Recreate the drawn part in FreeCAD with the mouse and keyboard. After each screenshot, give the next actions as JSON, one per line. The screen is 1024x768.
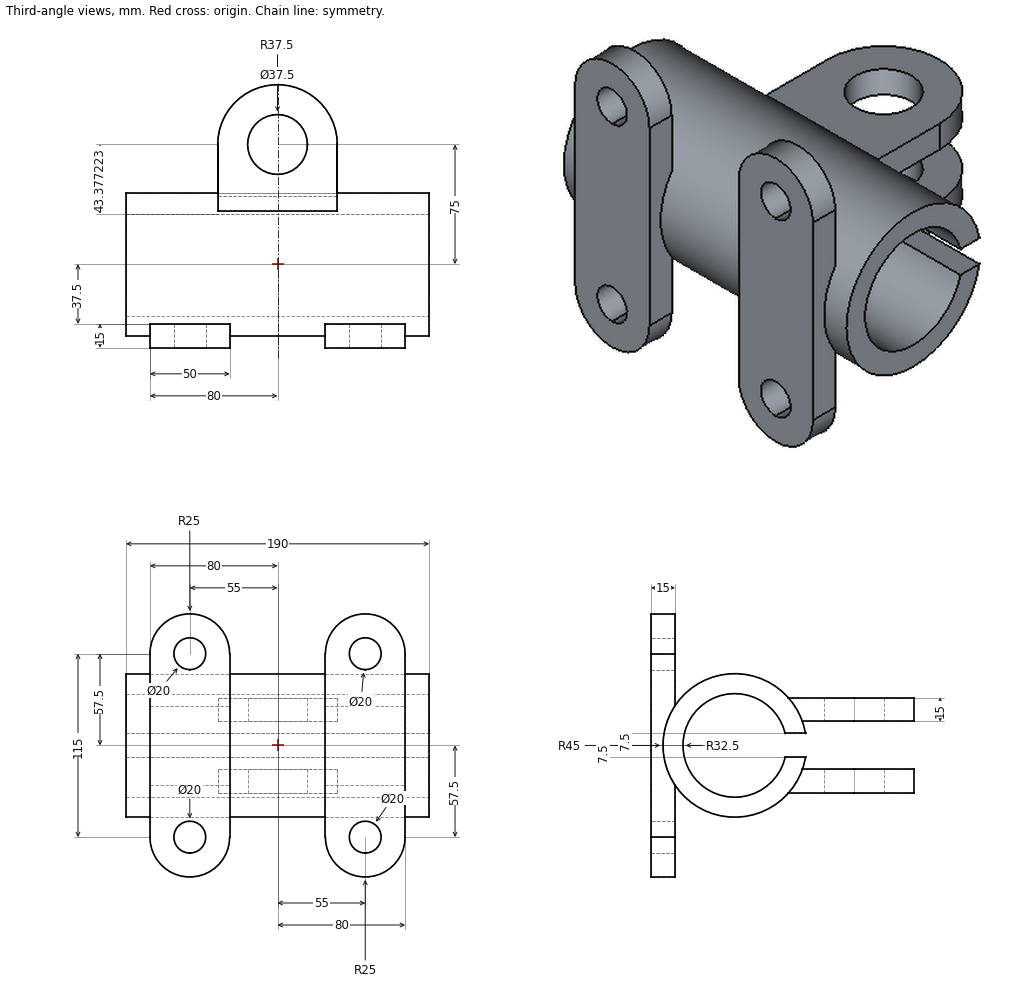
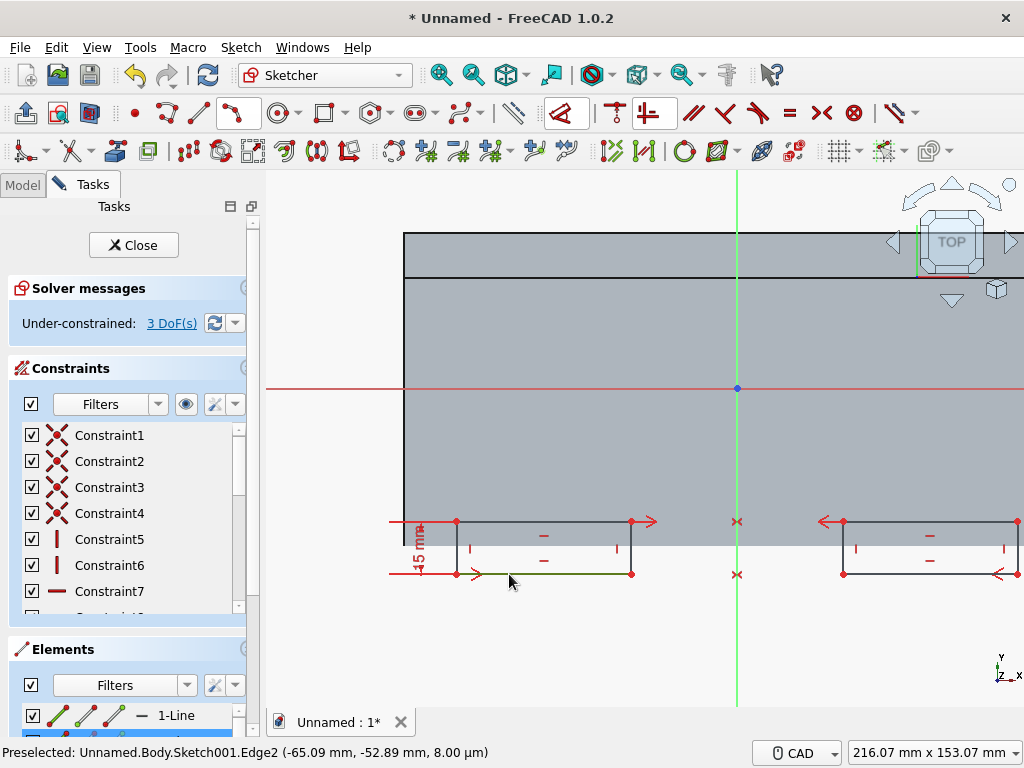
{"action": "left_click", "coordinate": [584, 114]}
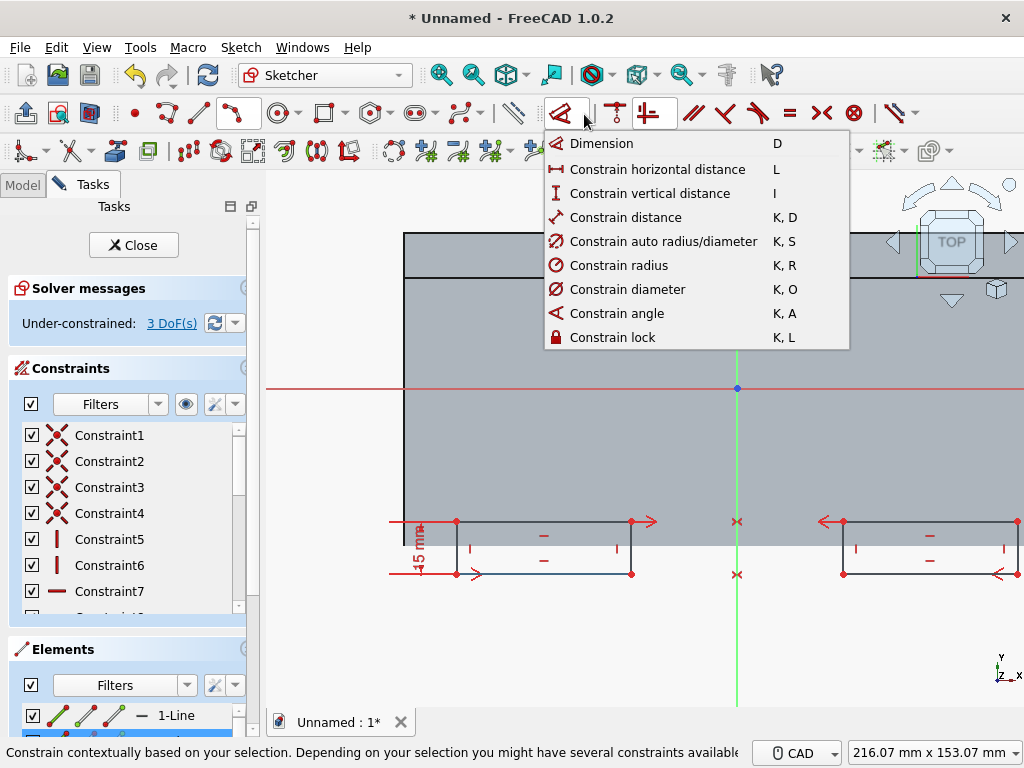
{"action": "left_click", "coordinate": [697, 169]}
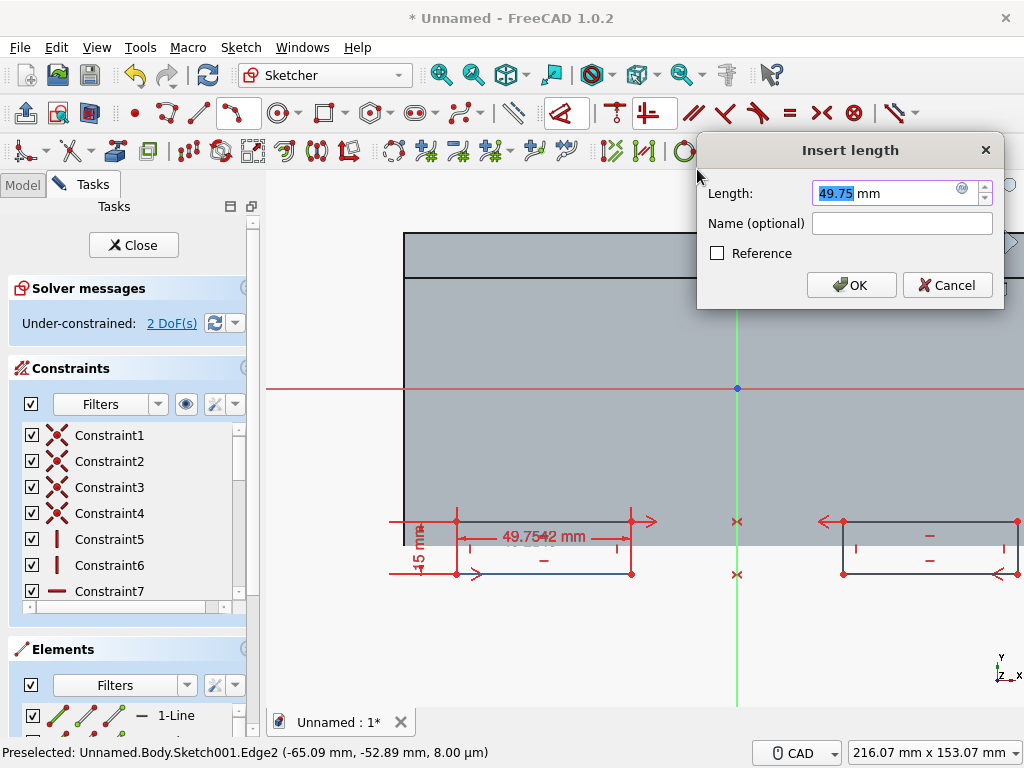
{"action": "type", "text": "50"}
{"action": "key", "text": "Return"}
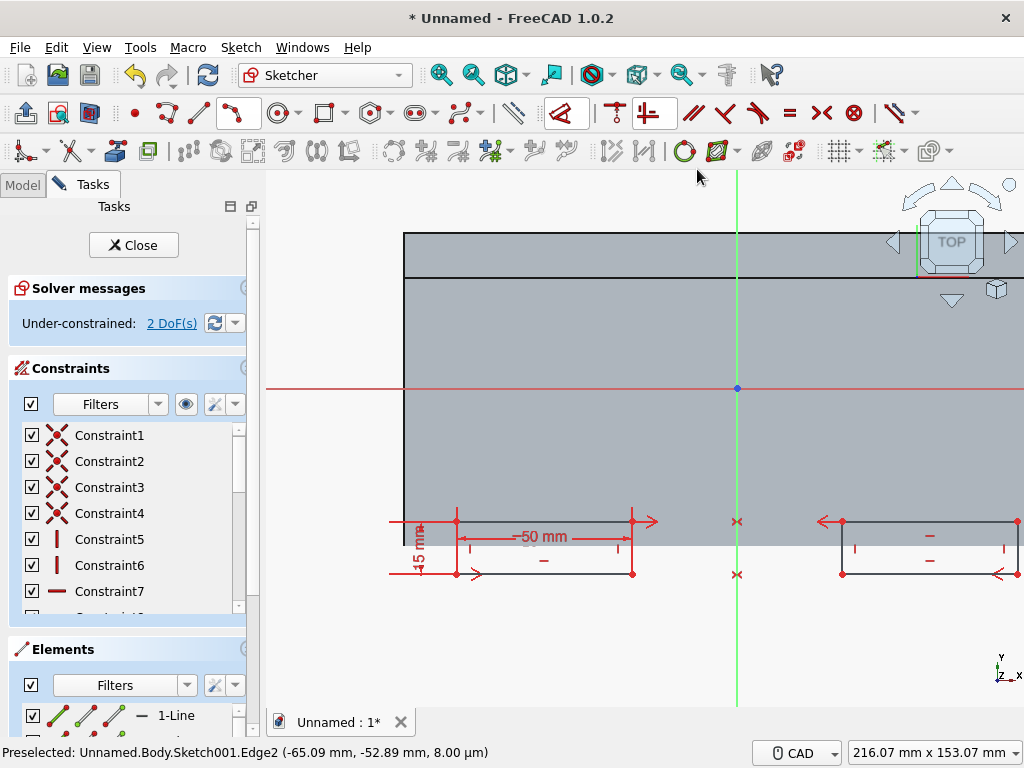
{"action": "left_click", "coordinate": [457, 522]}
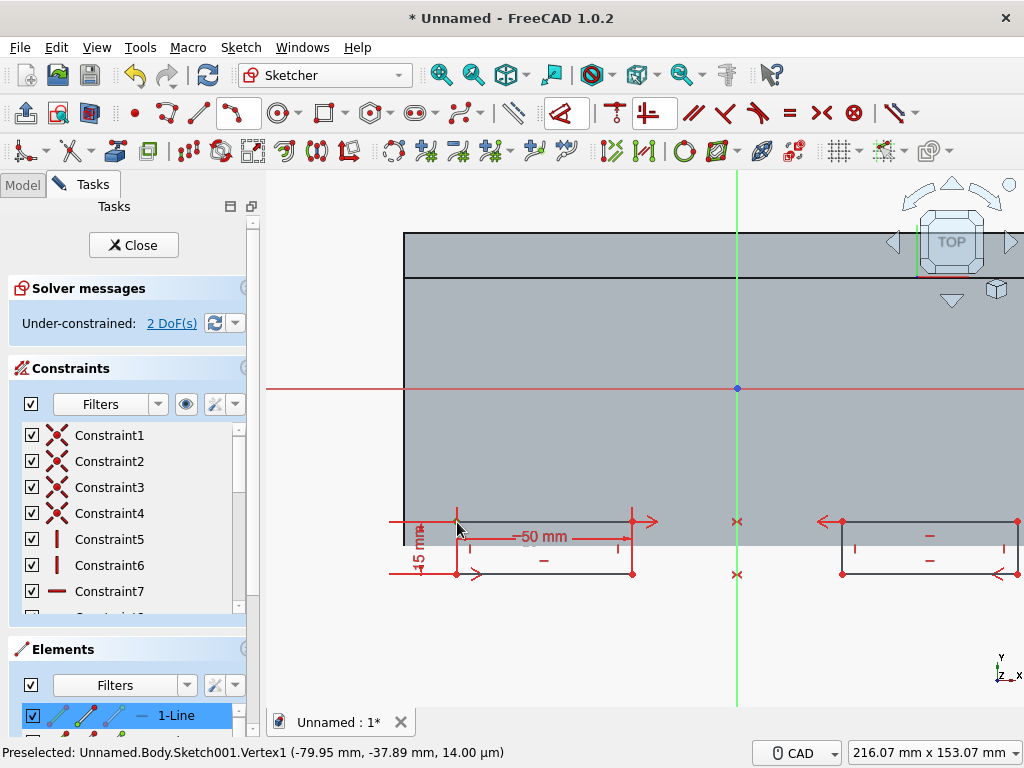
{"action": "left_click", "coordinate": [584, 114]}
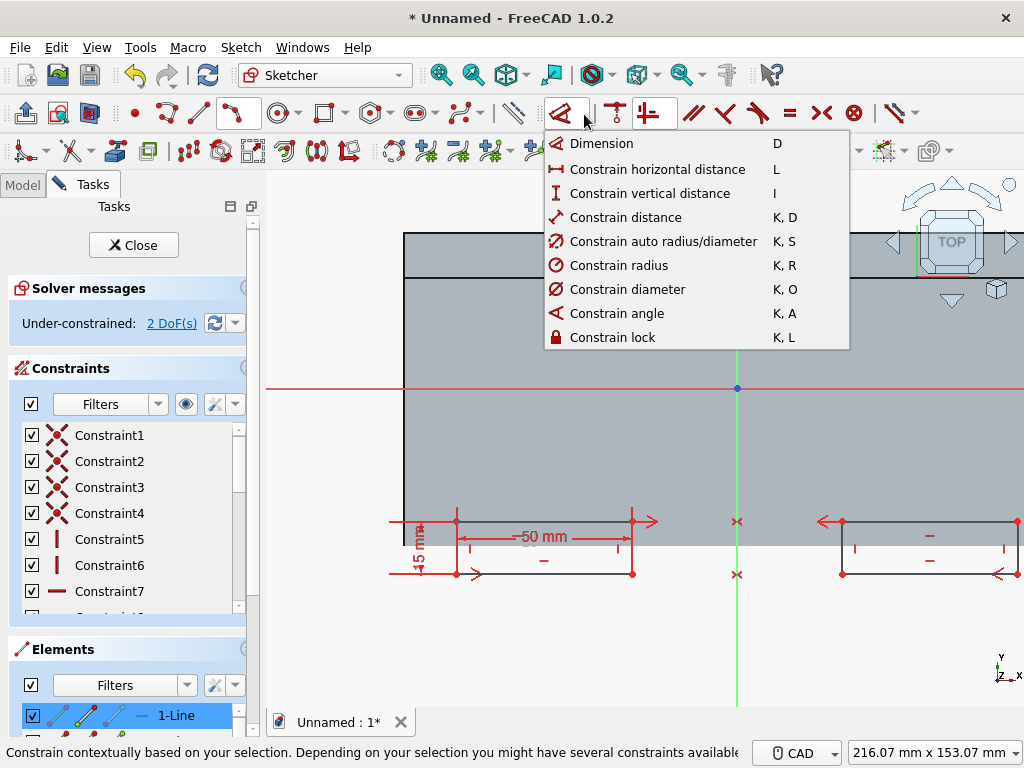
{"action": "left_click", "coordinate": [697, 169]}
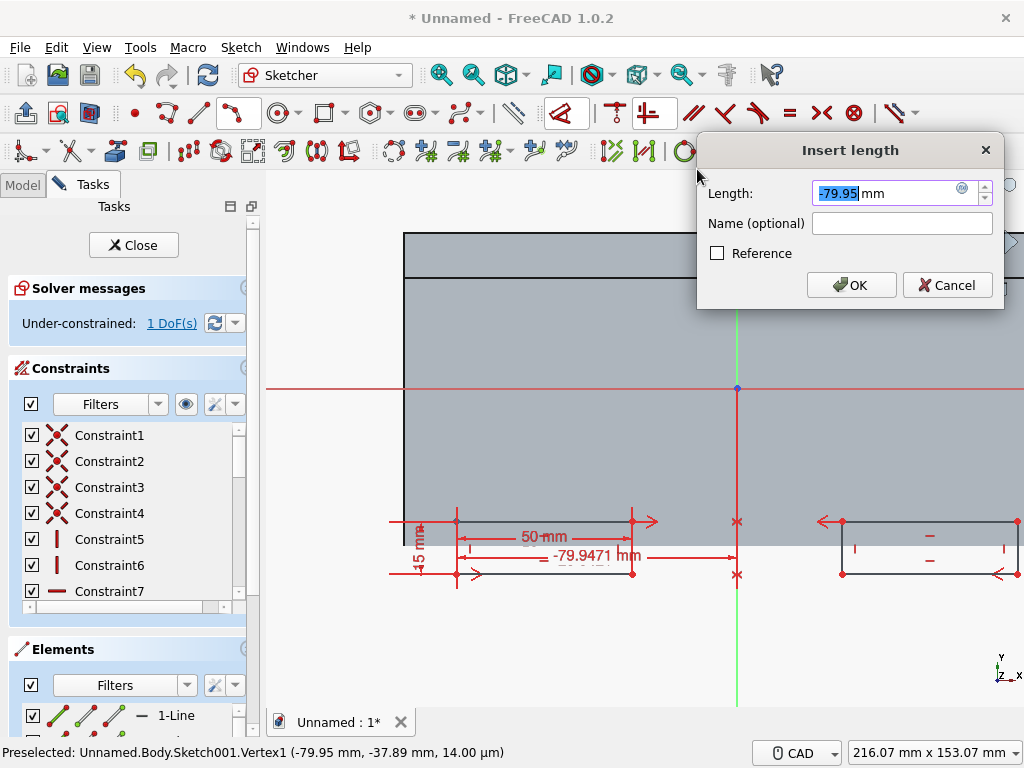
{"action": "type", "text": "-80"}
{"action": "key", "text": "Return"}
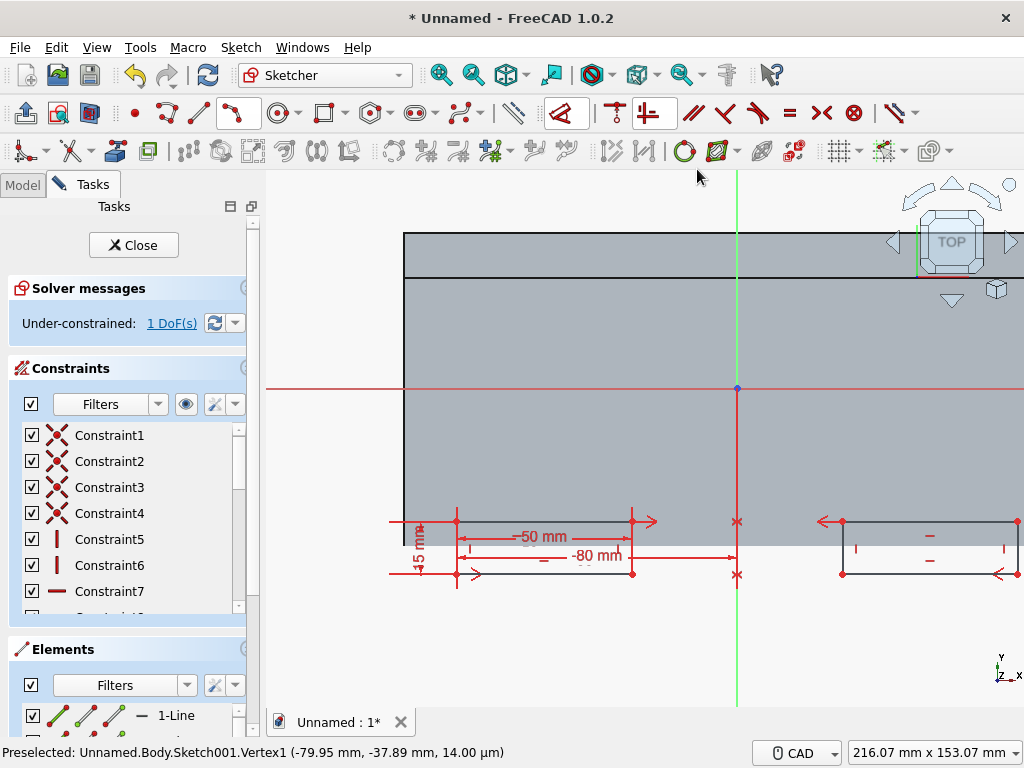
{"action": "left_click", "coordinate": [457, 522]}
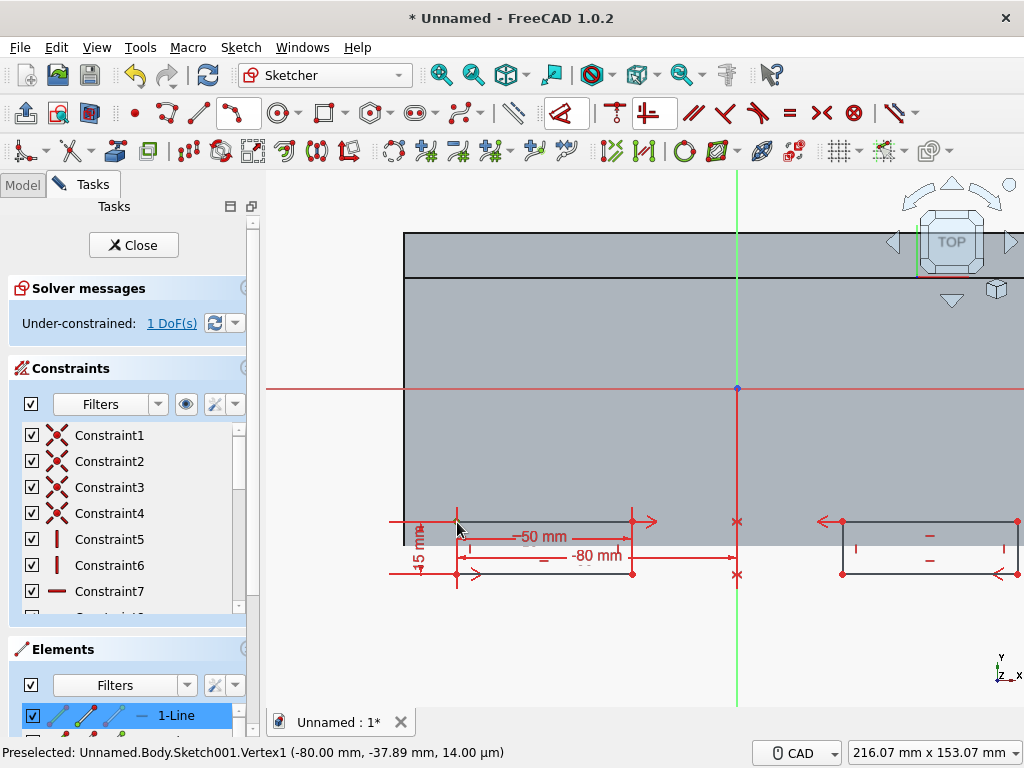
{"action": "left_click", "coordinate": [584, 114]}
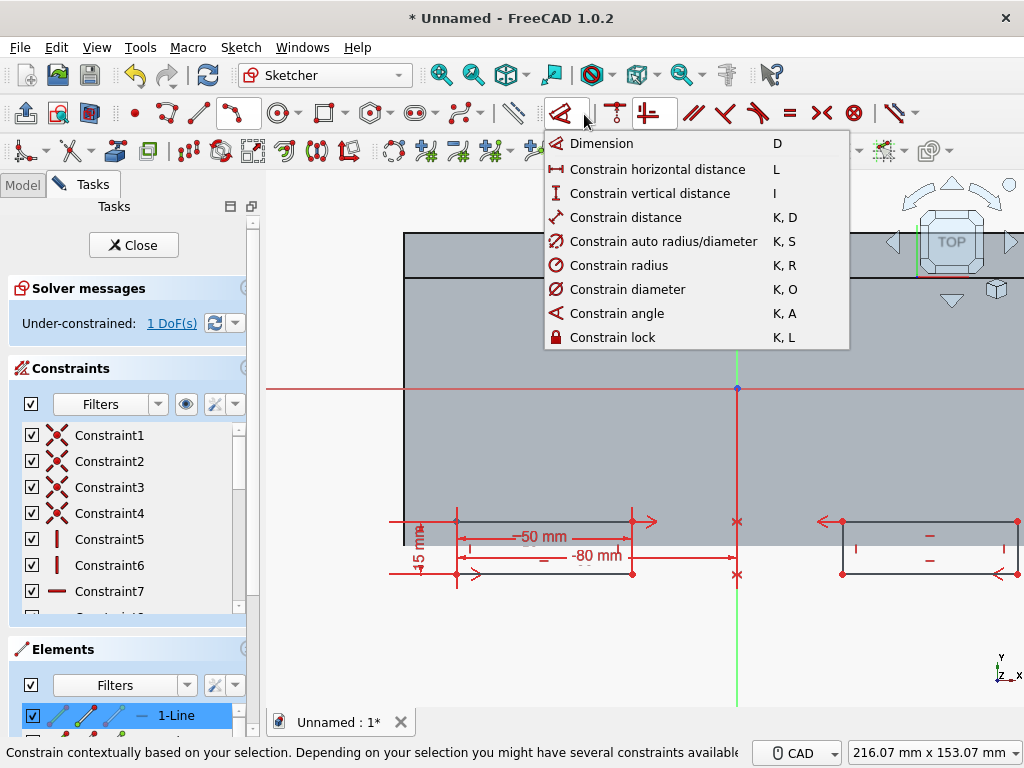
{"action": "left_click", "coordinate": [697, 193]}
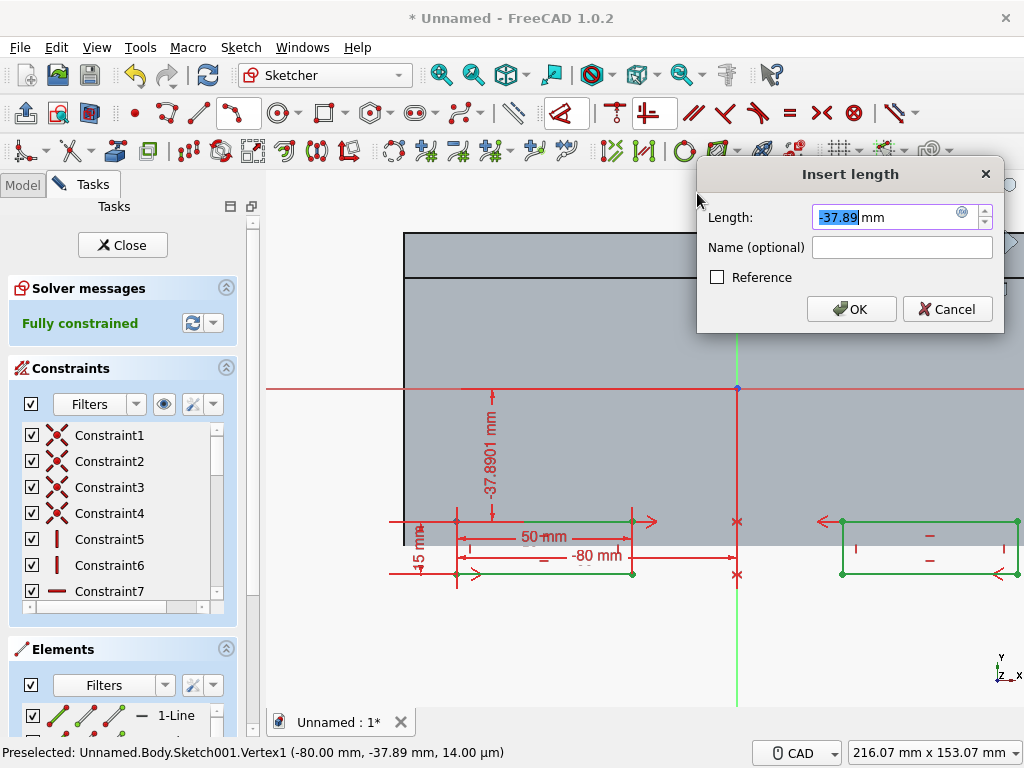
{"action": "type", "text": "-37.5"}
{"action": "key", "text": "Return"}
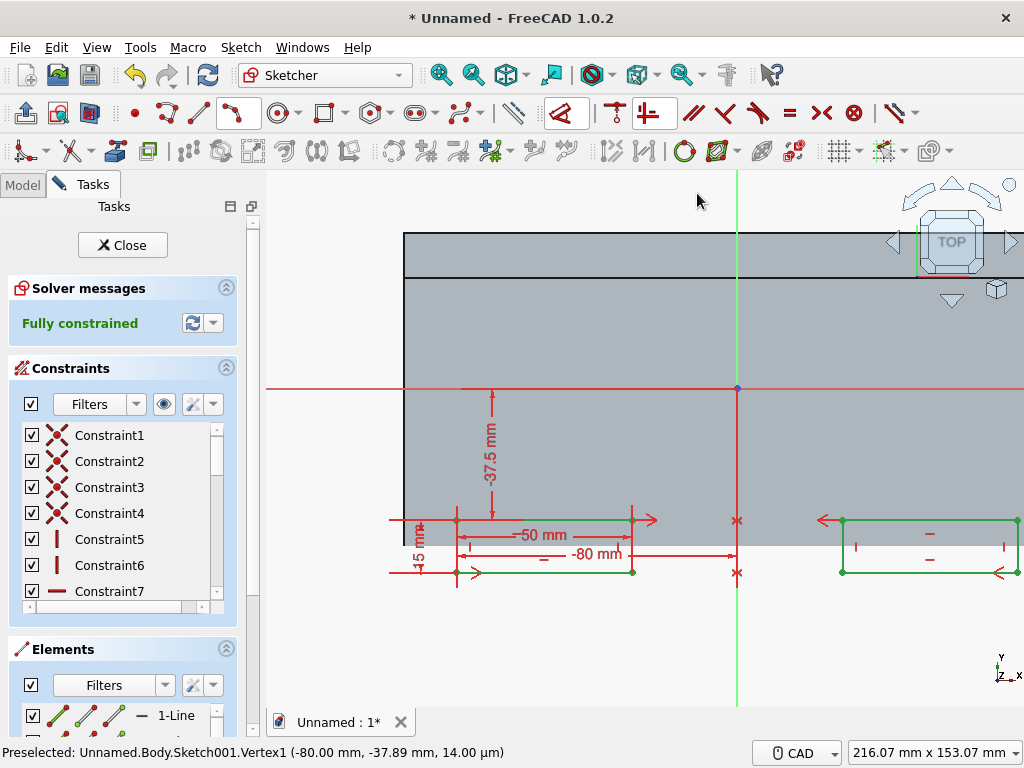
{"action": "left_click", "coordinate": [123, 245]}